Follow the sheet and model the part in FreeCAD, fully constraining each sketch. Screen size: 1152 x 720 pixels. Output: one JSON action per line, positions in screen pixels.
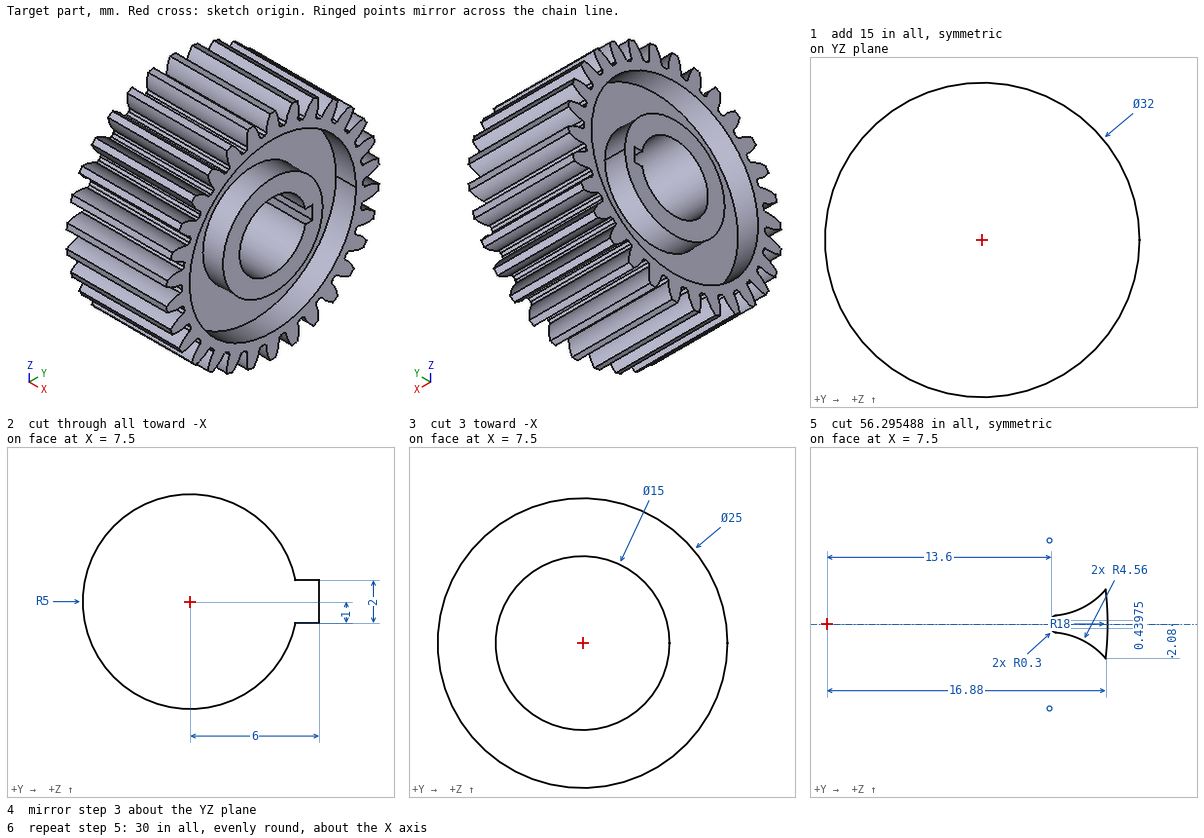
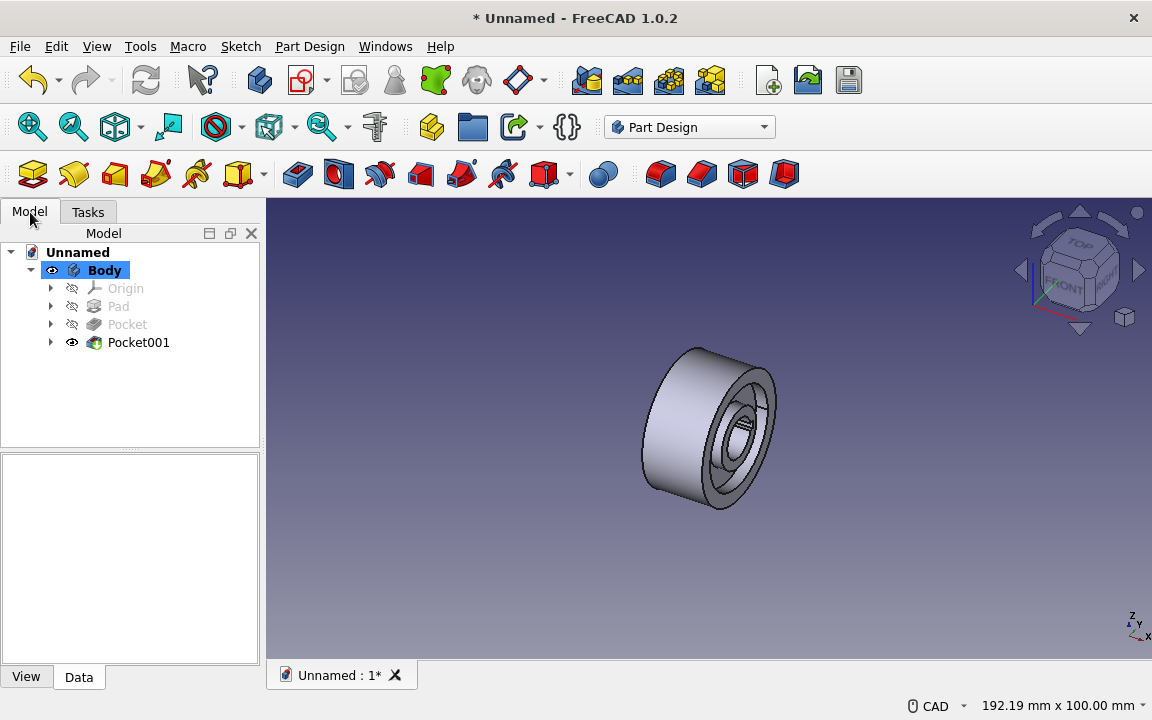
{"action": "left_click", "coordinate": [117, 342]}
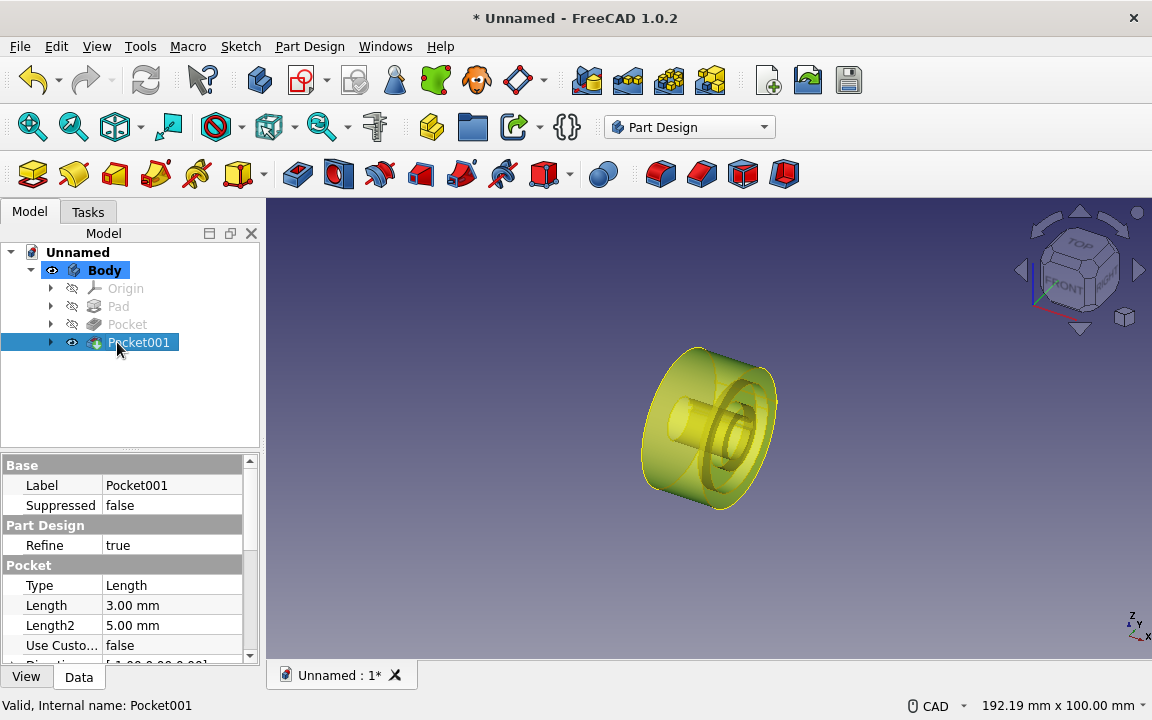
{"action": "left_click", "coordinate": [587, 80]}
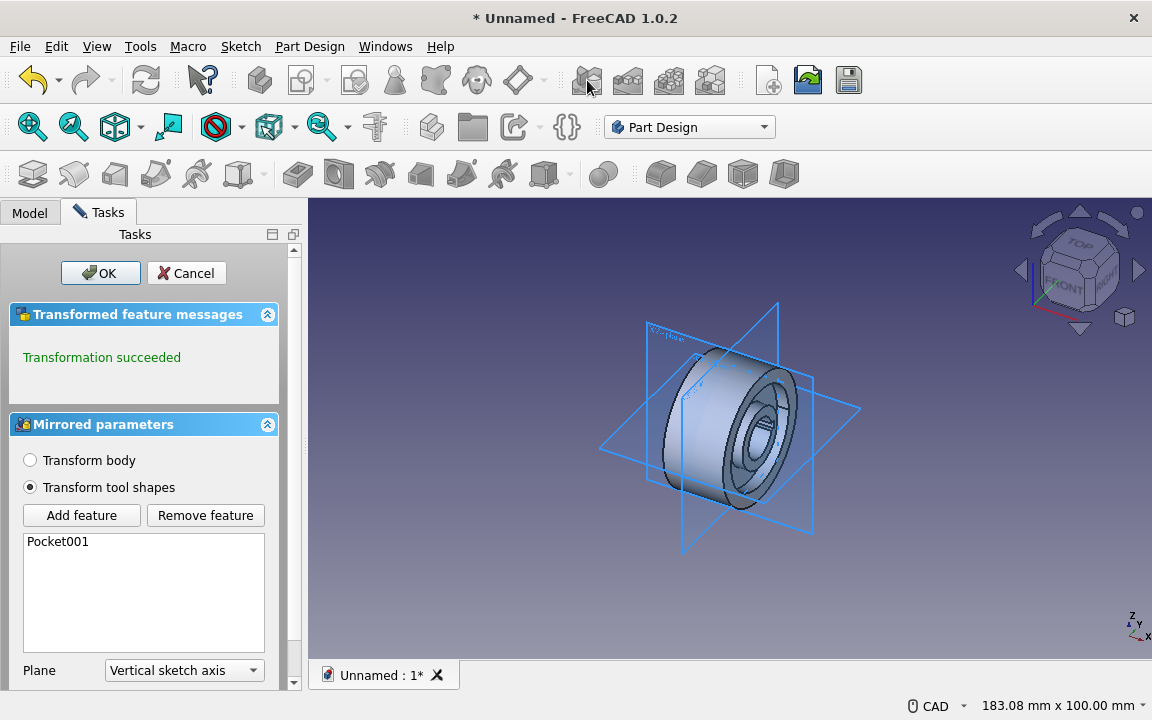
{"action": "left_click", "coordinate": [185, 670]}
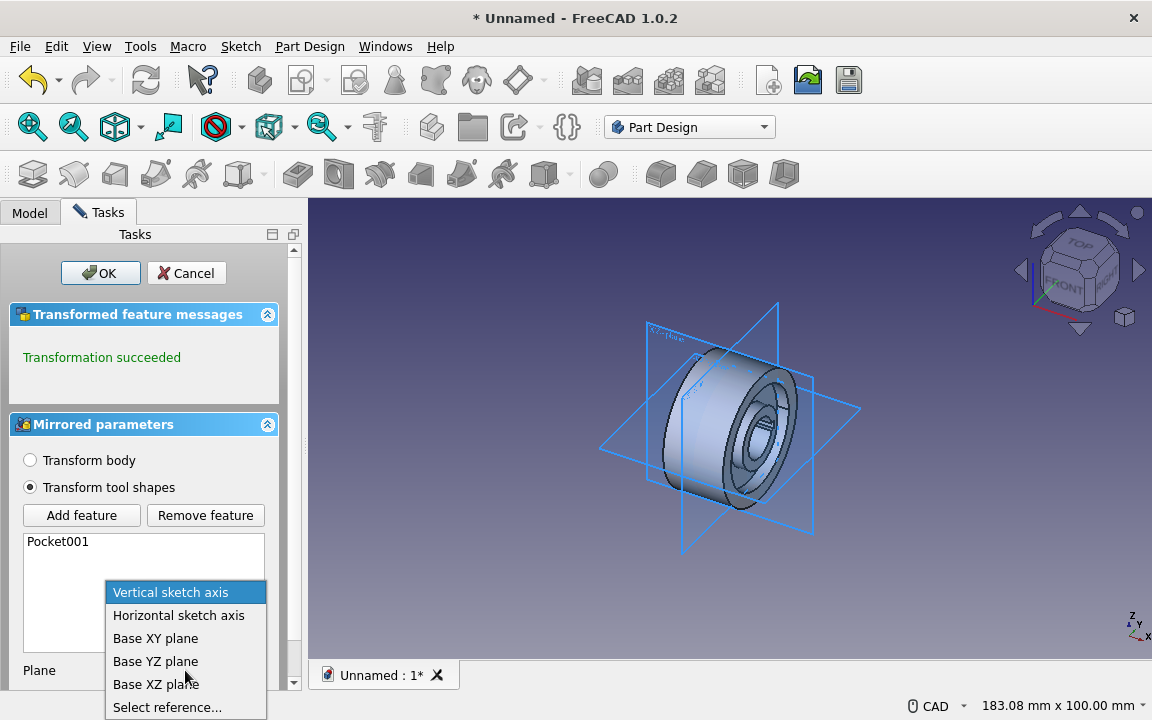
{"action": "left_click", "coordinate": [184, 662]}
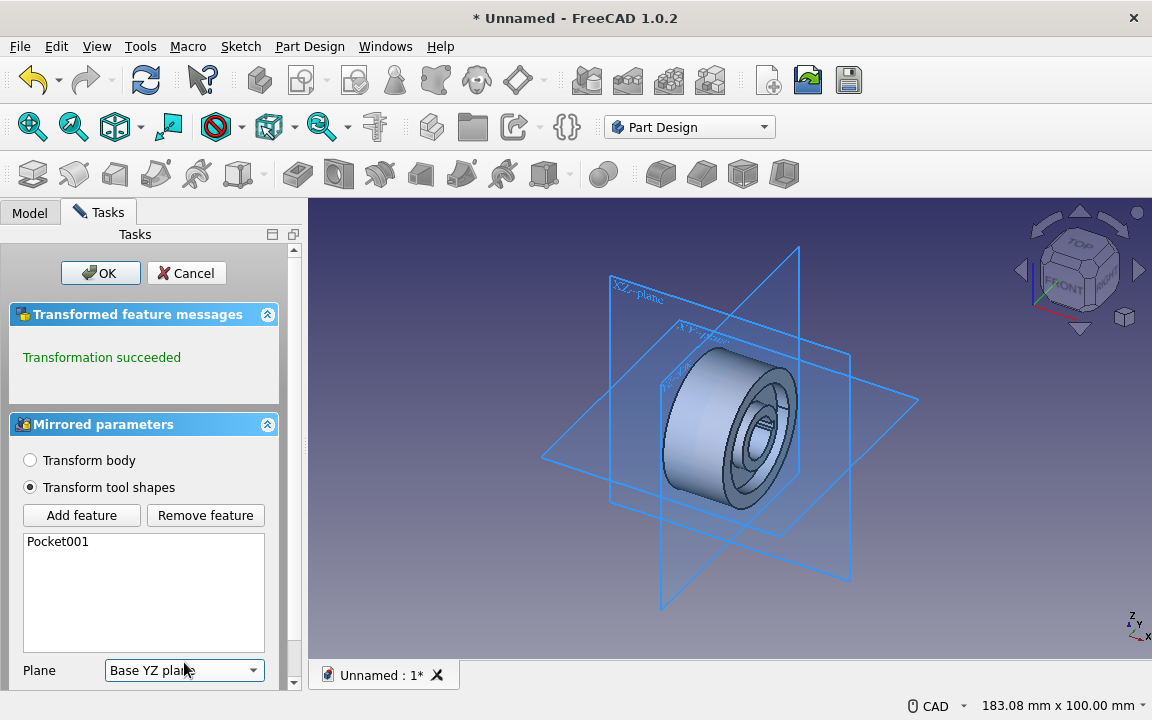
{"action": "left_click", "coordinate": [101, 273]}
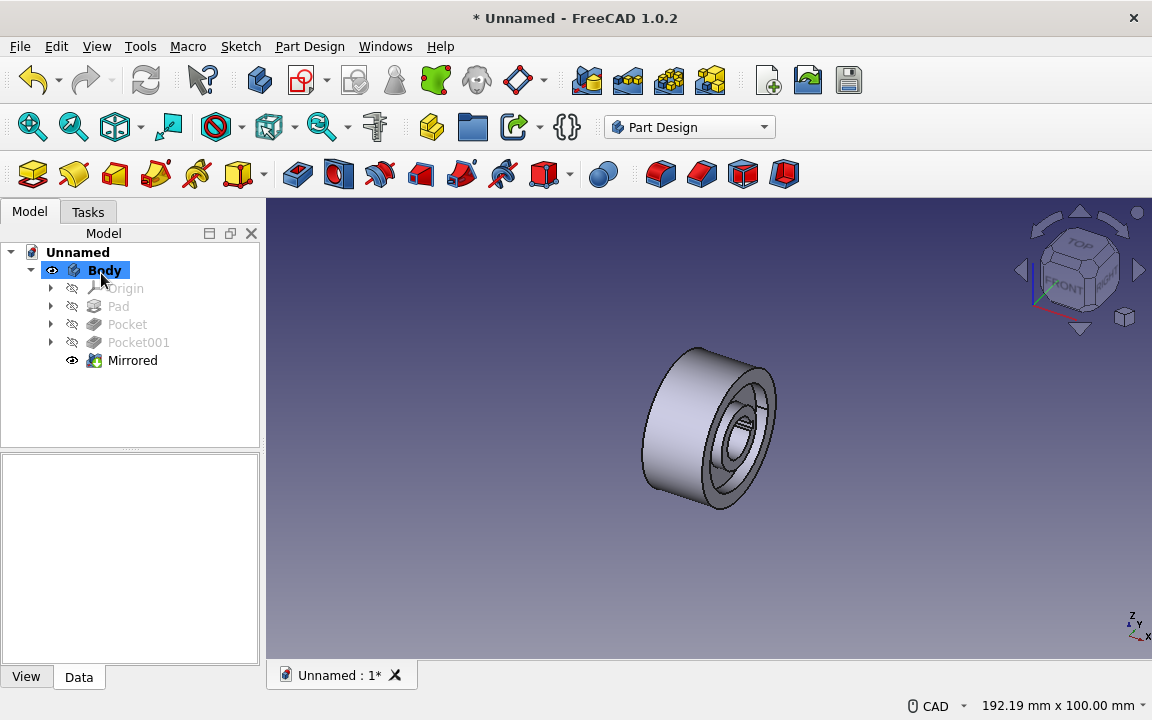
{"action": "key", "text": "0"}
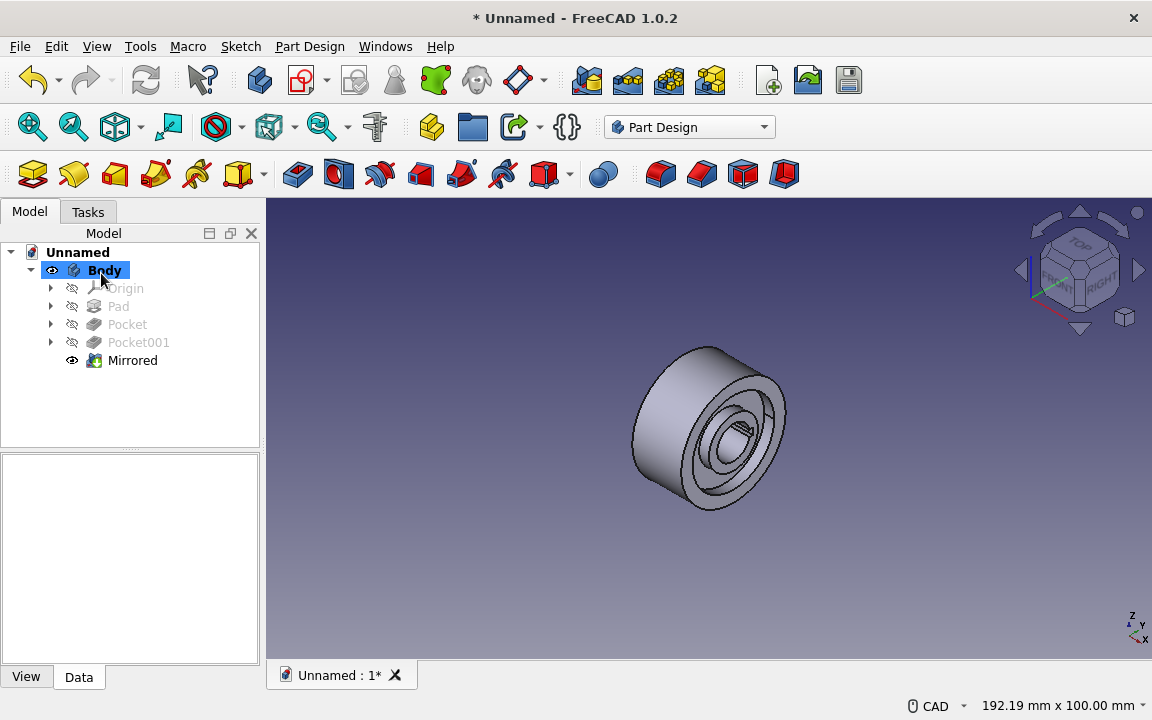
{"action": "key", "text": "3"}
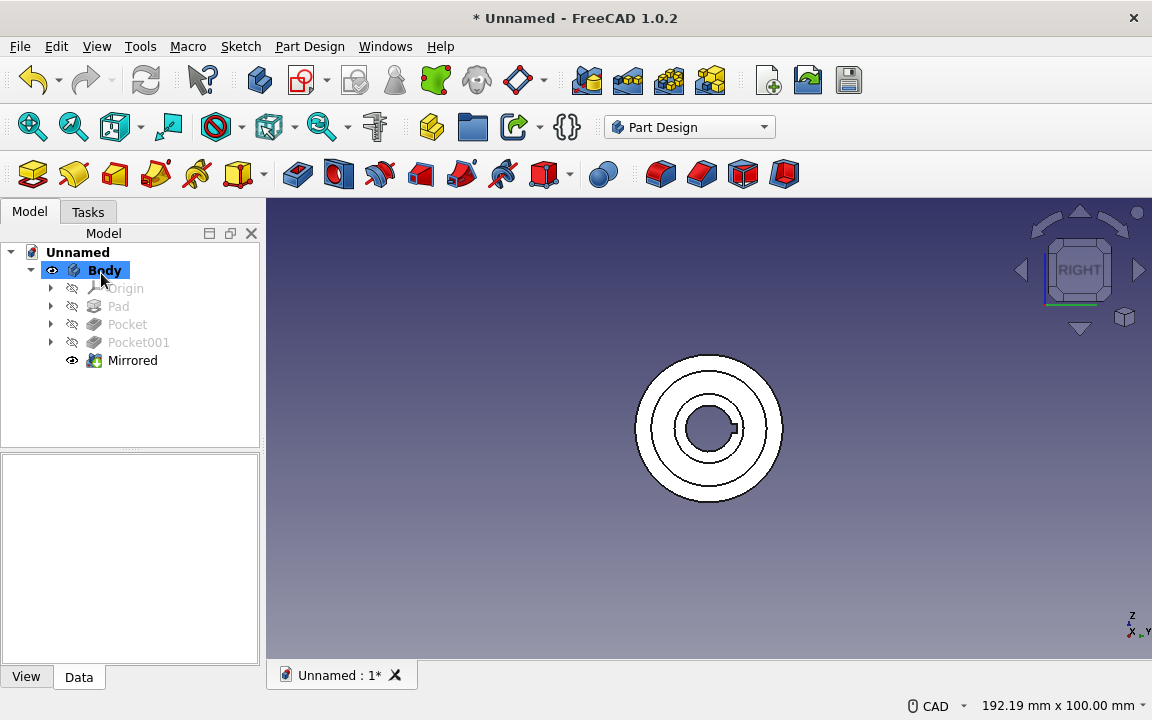
{"action": "key", "text": "v f"}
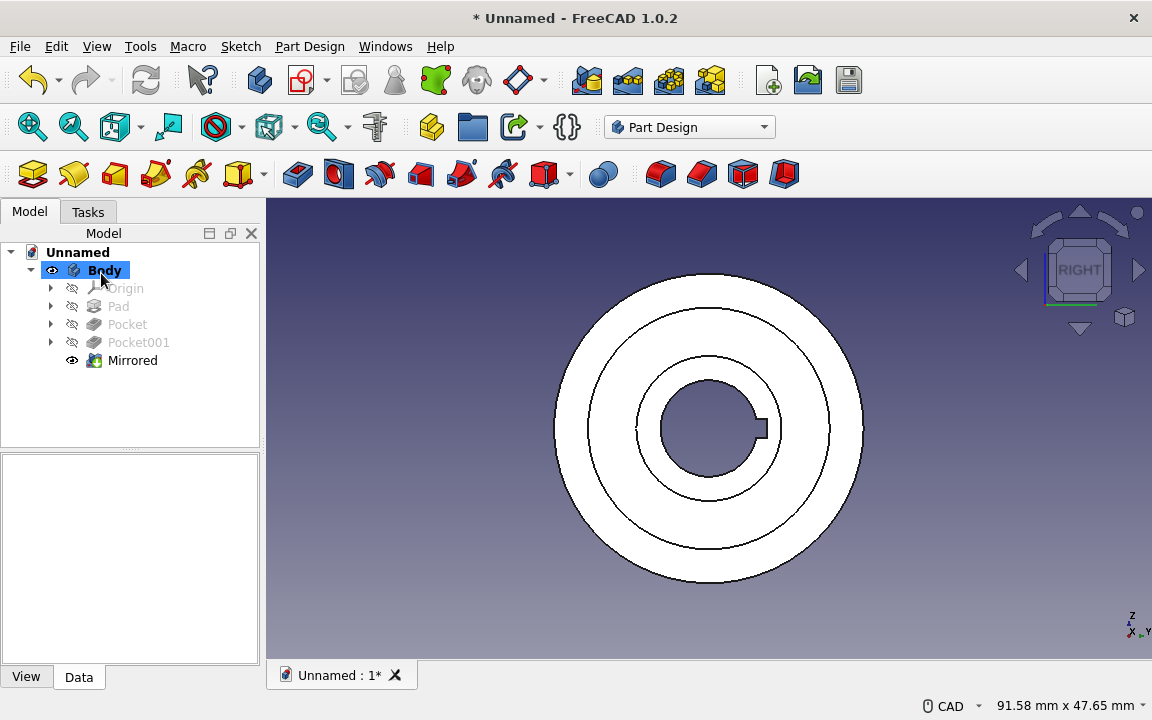
{"action": "left_click", "coordinate": [842, 472]}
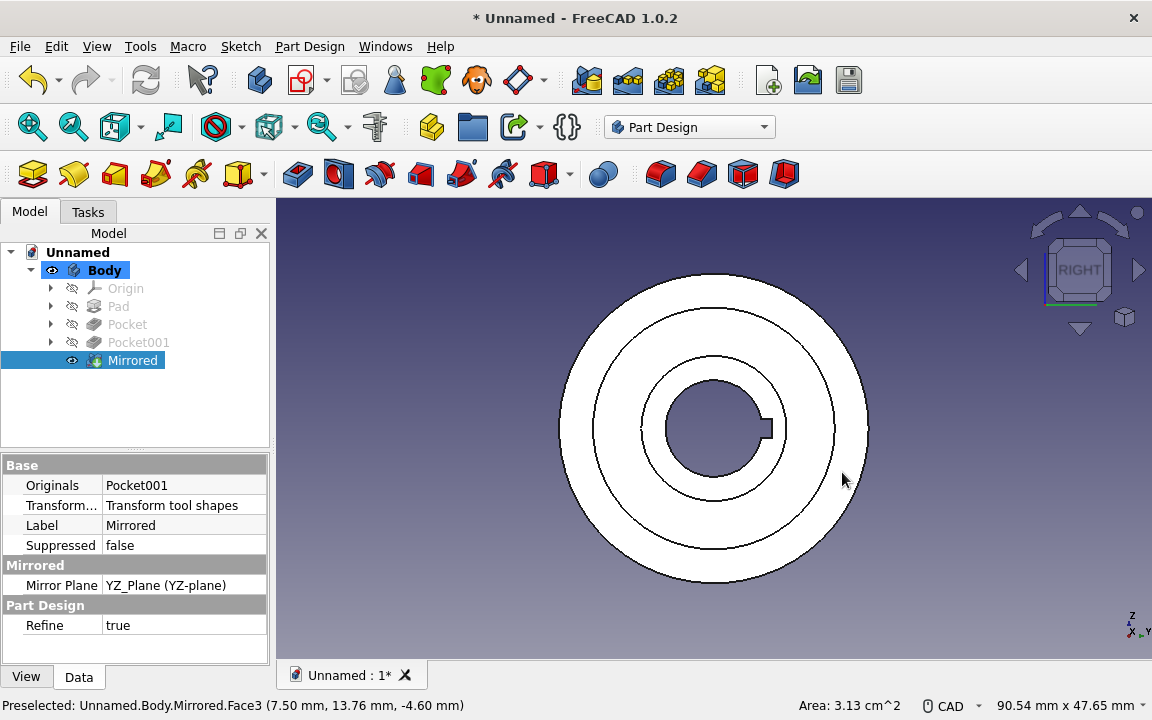
{"action": "left_click", "coordinate": [300, 80]}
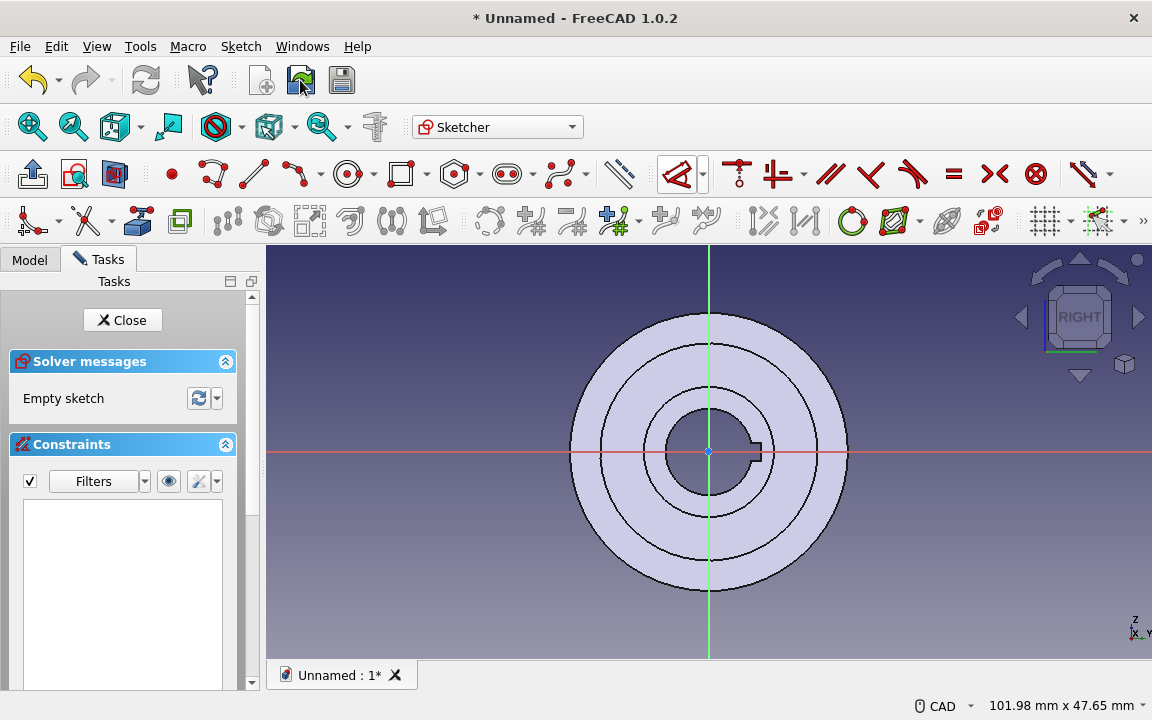
{"action": "scroll", "coordinate": [873, 452], "scroll_direction": "up", "scroll_amount": 10}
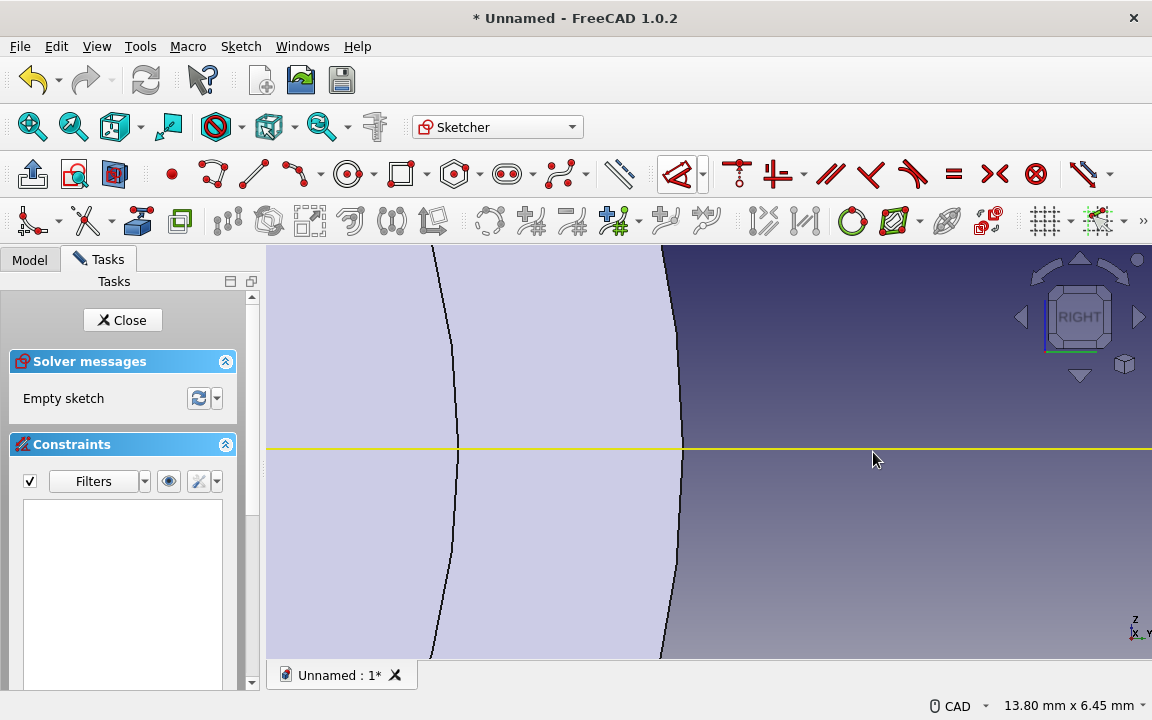
{"action": "key", "text": "g l"}